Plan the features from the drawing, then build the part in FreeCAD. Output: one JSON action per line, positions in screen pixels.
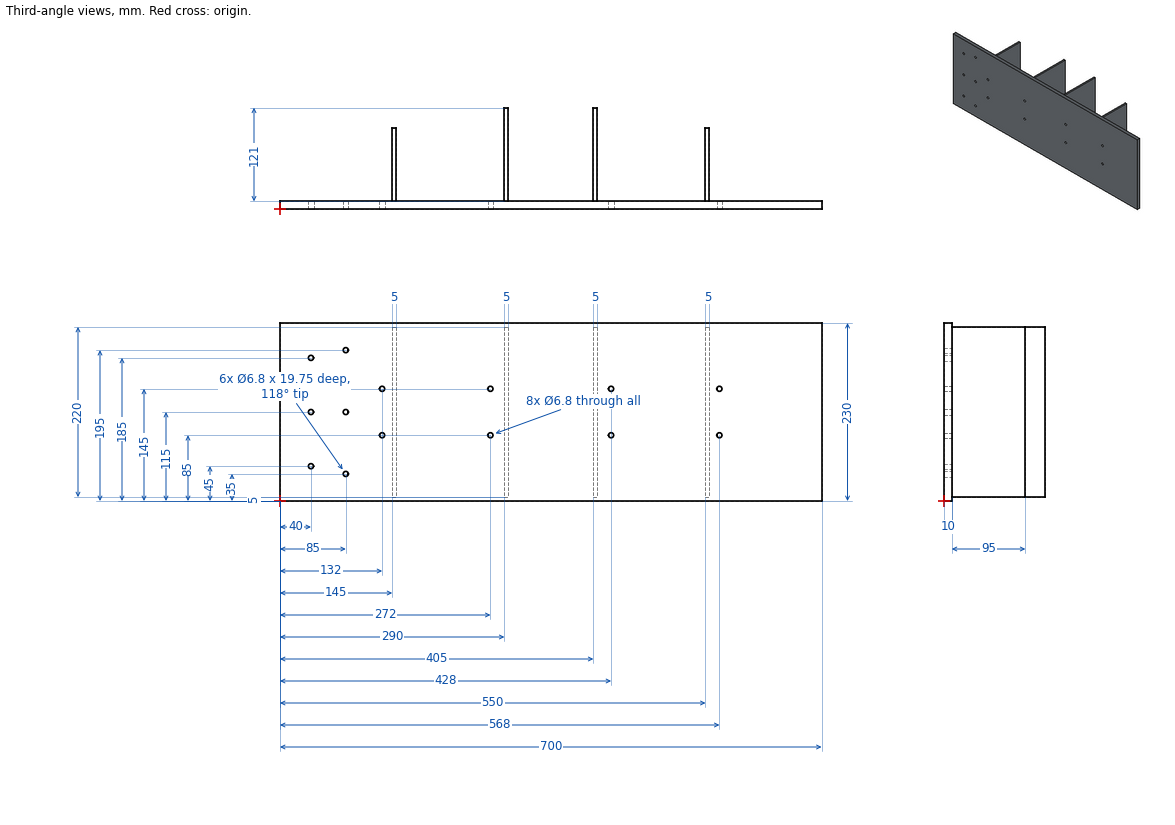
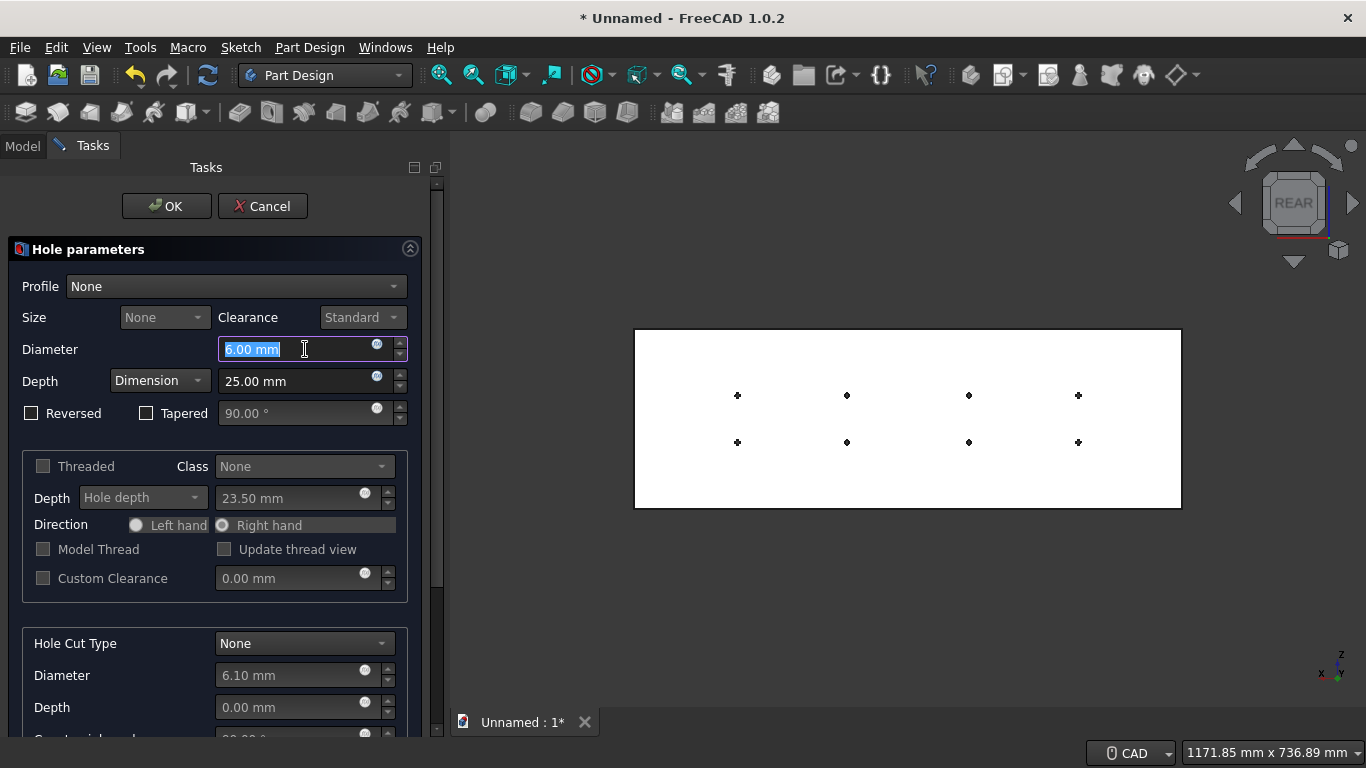
{"action": "type", "text": "6.8"}
{"action": "key", "text": "Tab"}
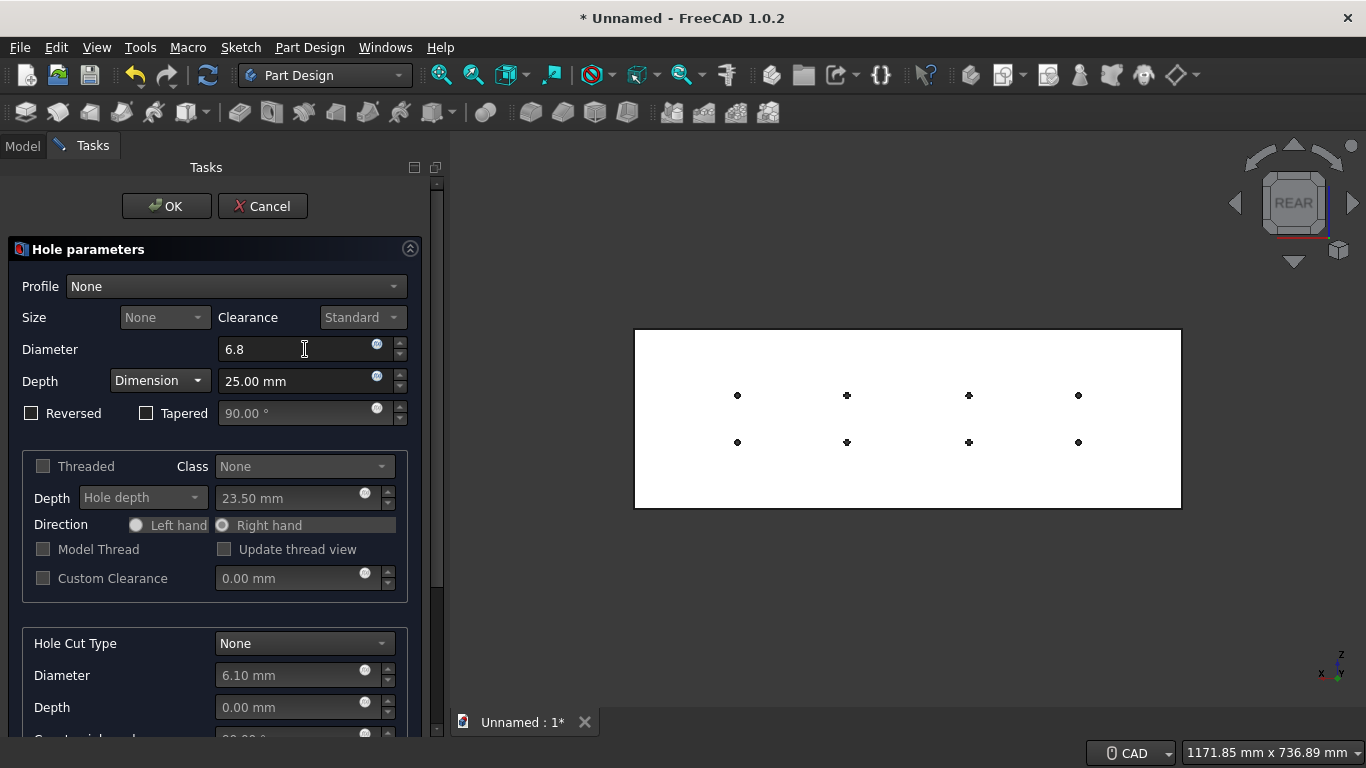
{"action": "left_click", "coordinate": [161, 380]}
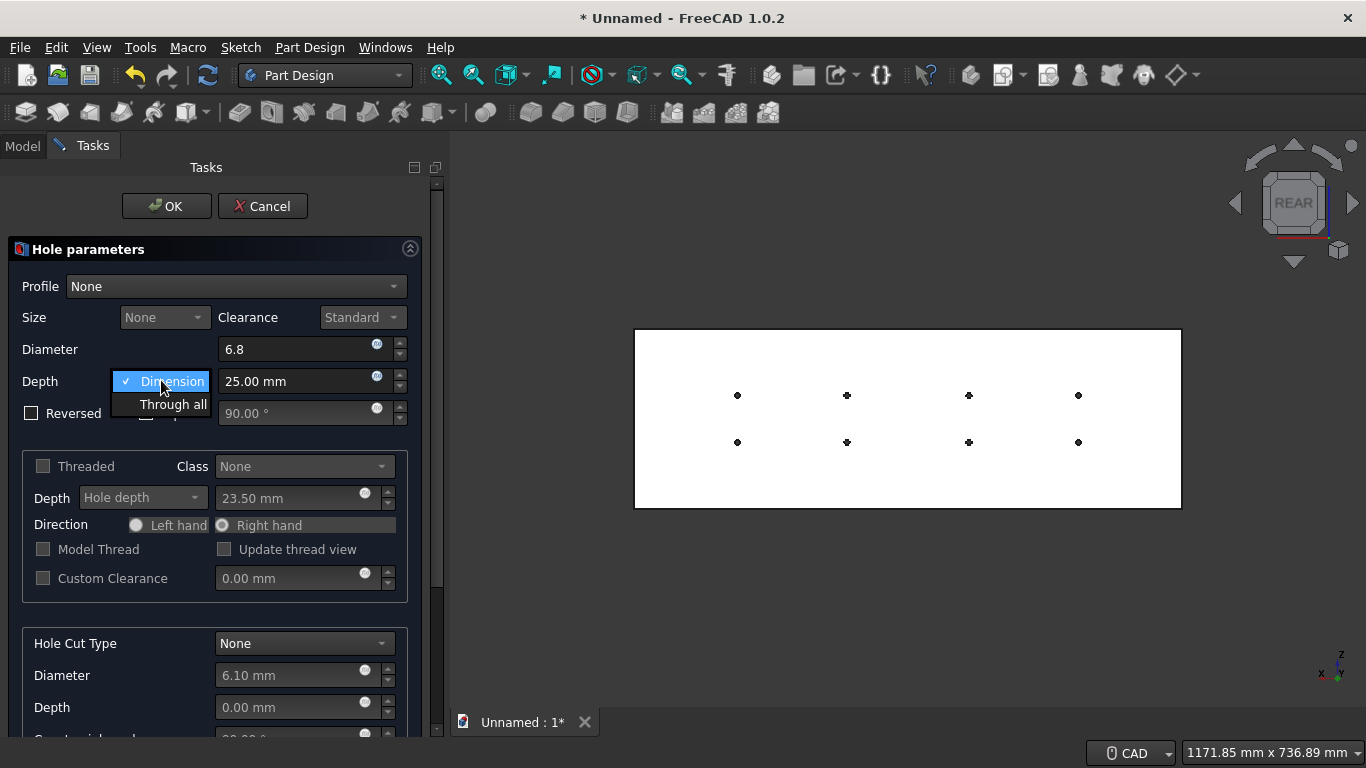
{"action": "left_click", "coordinate": [160, 404]}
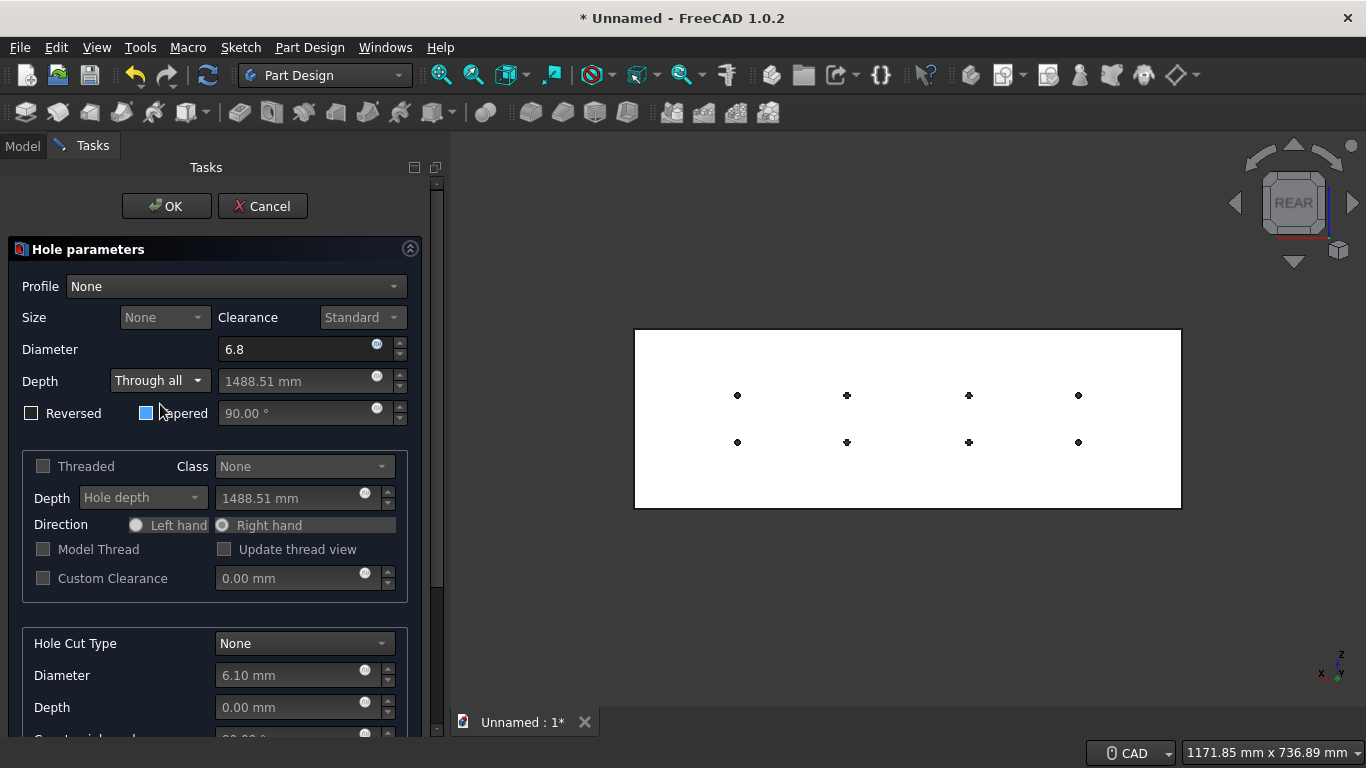
{"action": "left_click", "coordinate": [167, 206]}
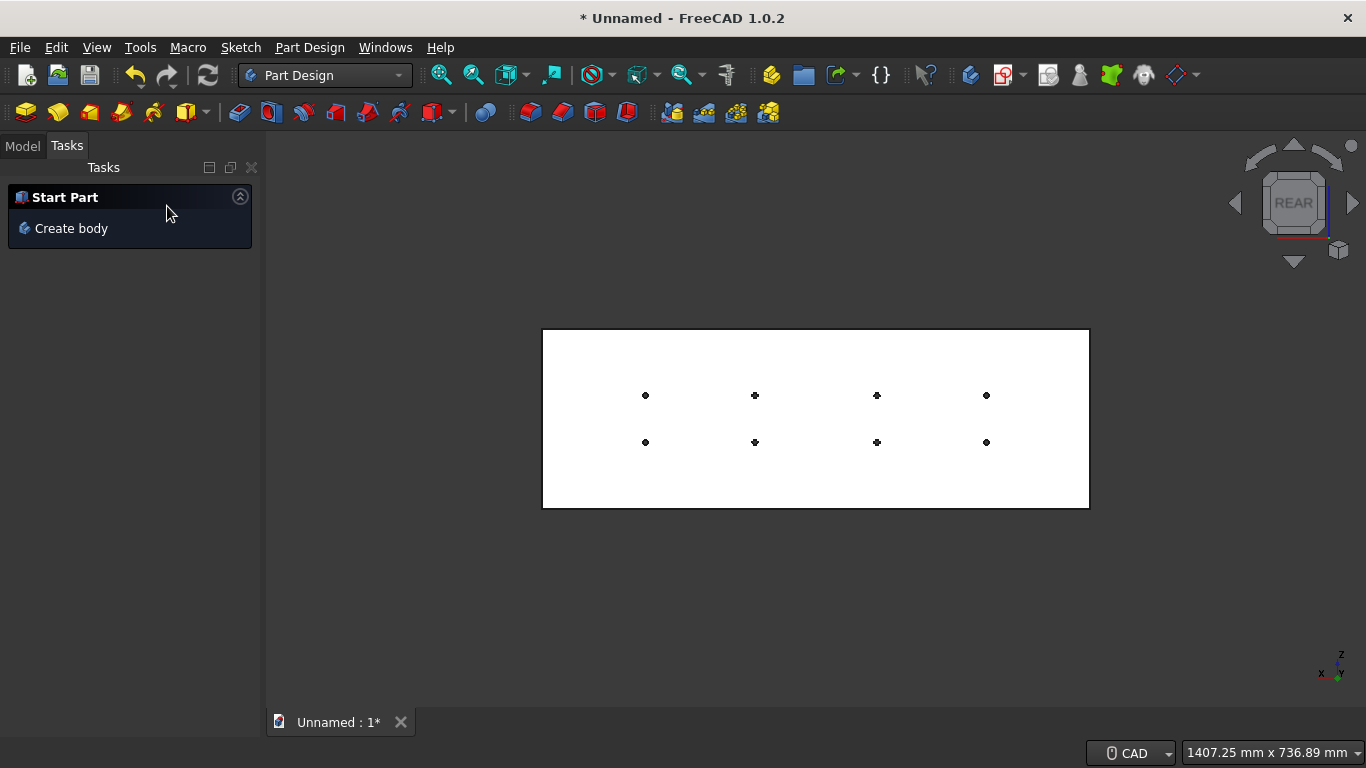
{"action": "left_click", "coordinate": [816, 418]}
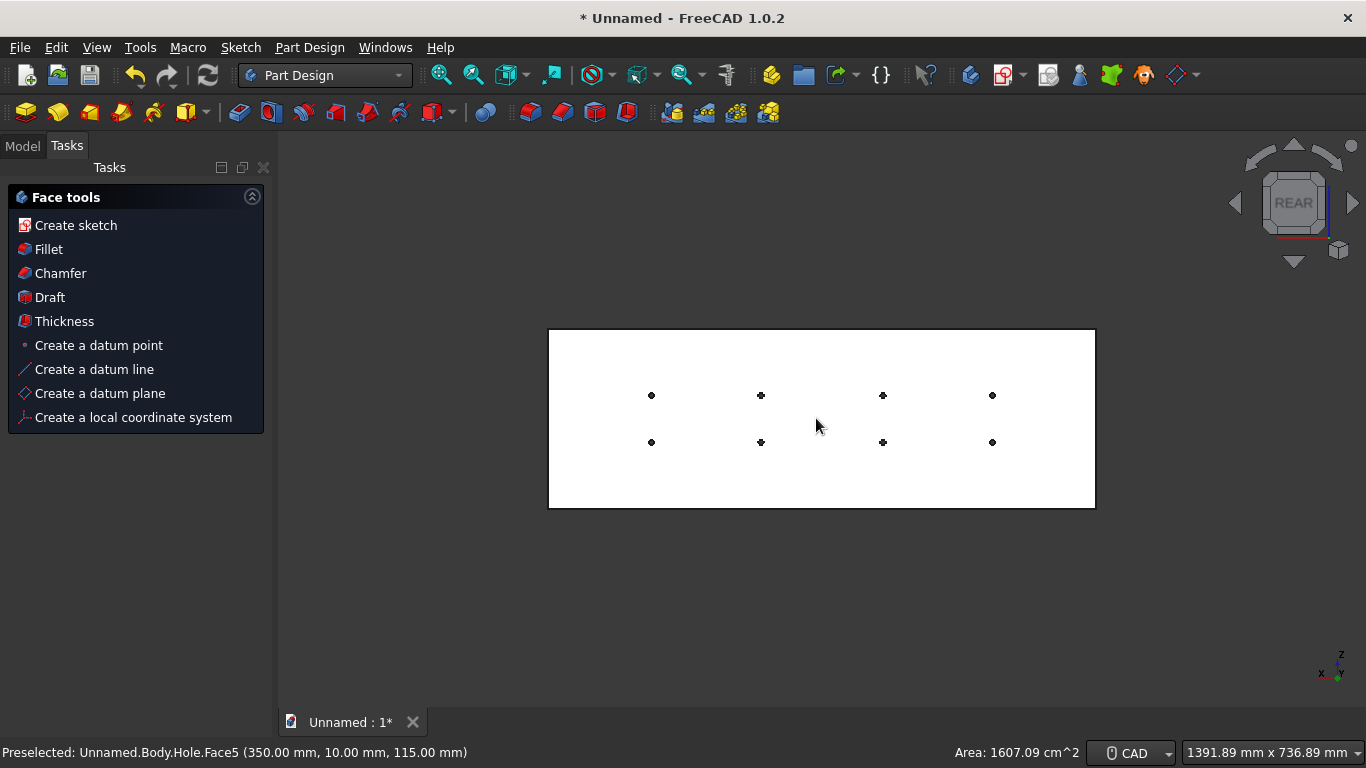
{"action": "left_click", "coordinate": [1004, 76]}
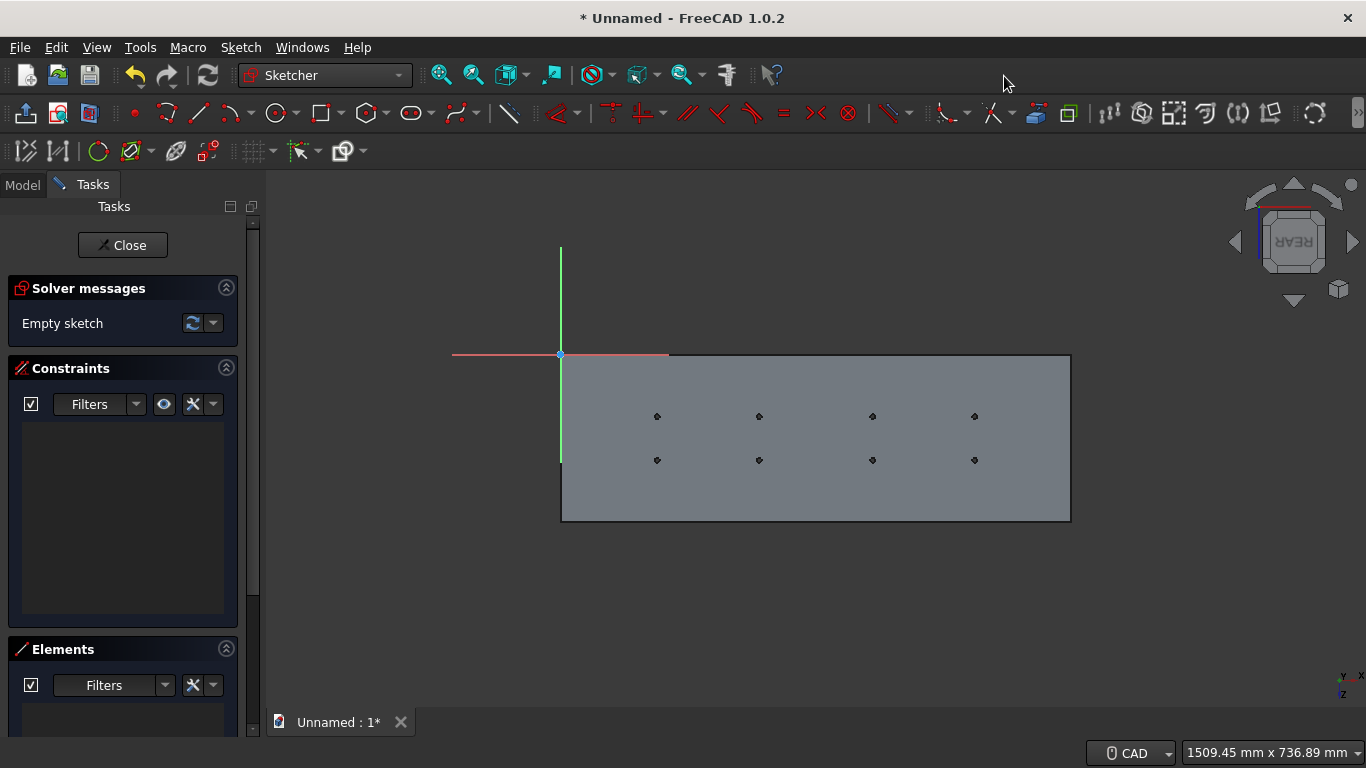
{"action": "scroll", "coordinate": [680, 435], "scroll_direction": "up", "scroll_amount": 4}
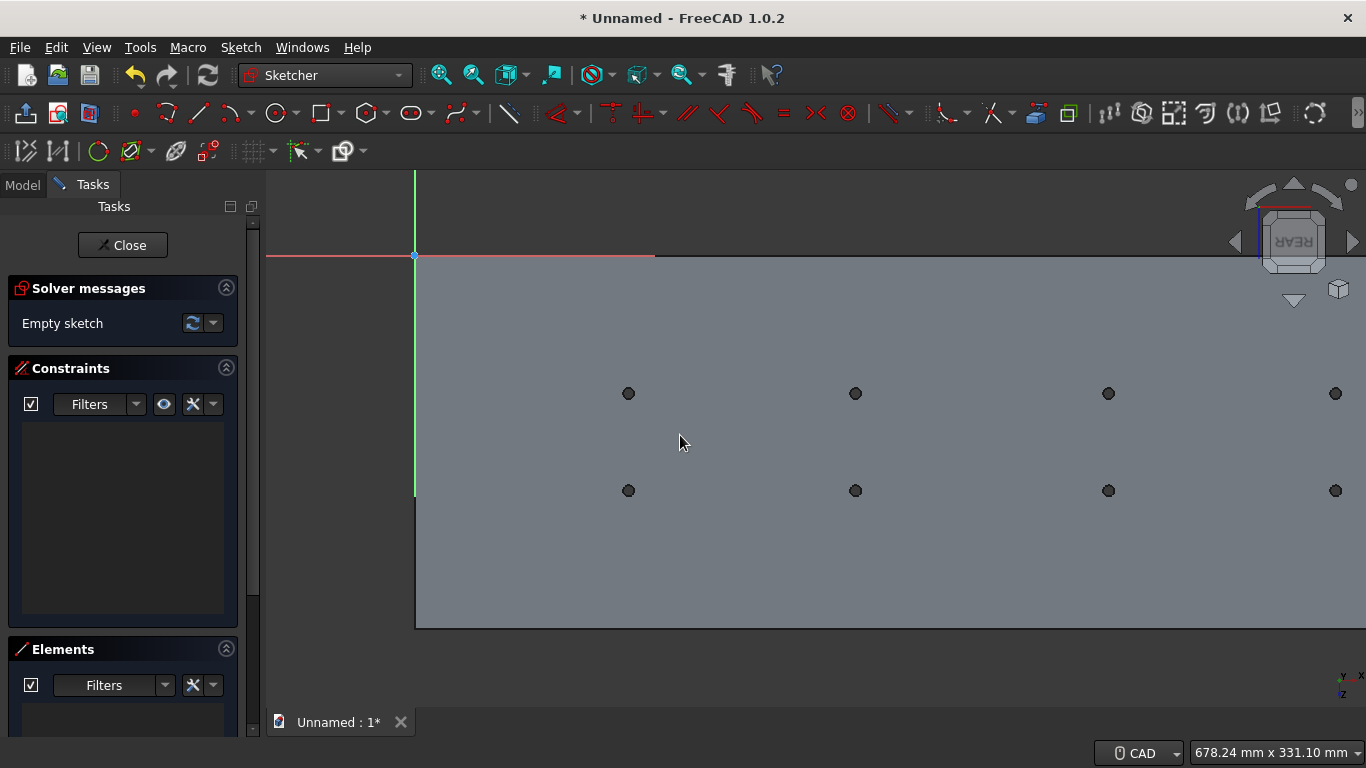
{"action": "key", "text": "g r"}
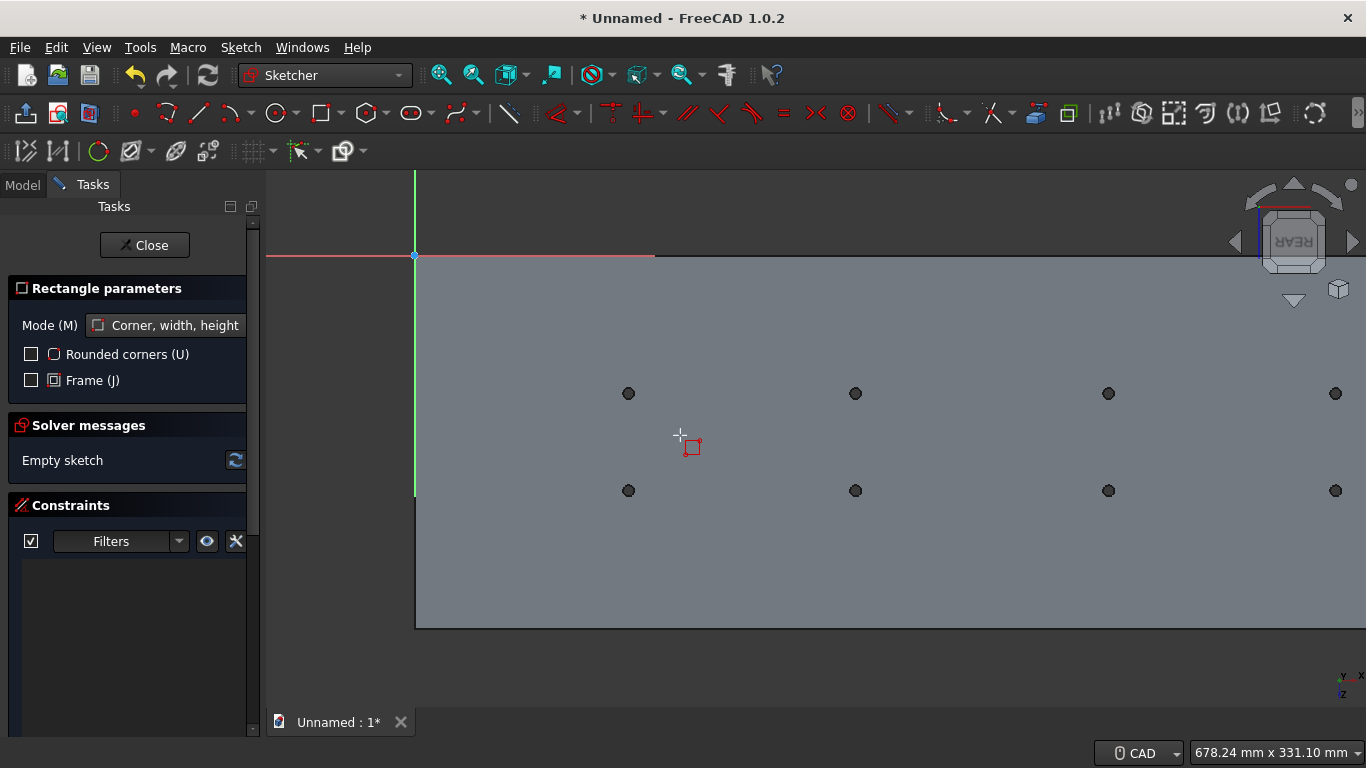
{"action": "scroll", "coordinate": [885, 264], "scroll_direction": "up", "scroll_amount": 4}